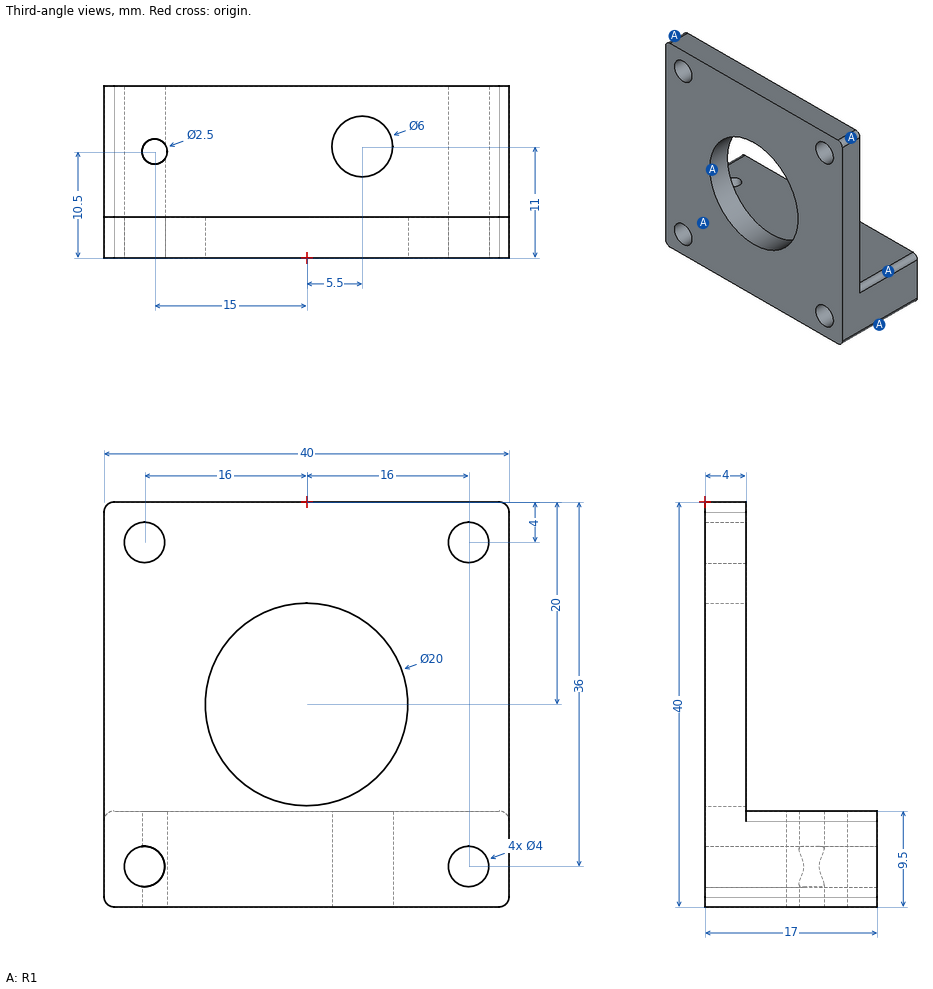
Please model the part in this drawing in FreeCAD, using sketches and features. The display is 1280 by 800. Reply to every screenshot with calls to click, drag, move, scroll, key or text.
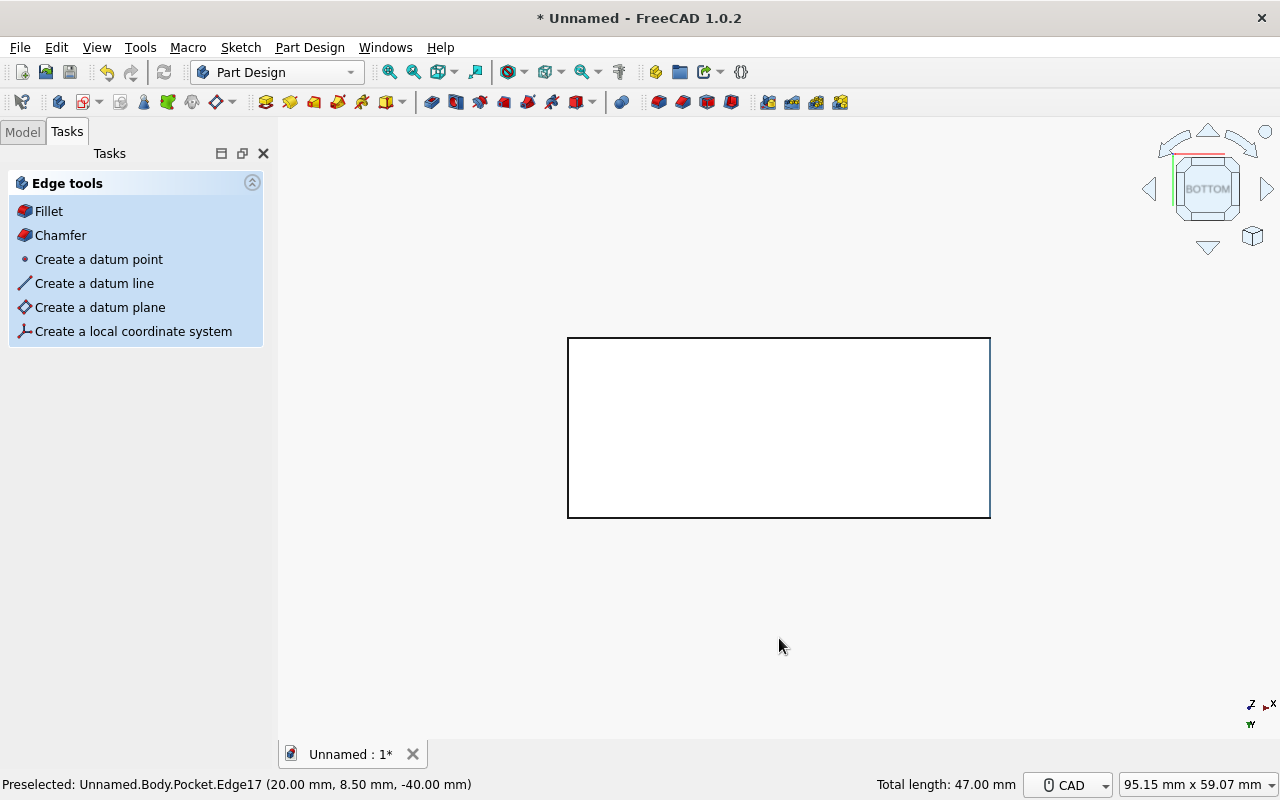
key(v)
key(f)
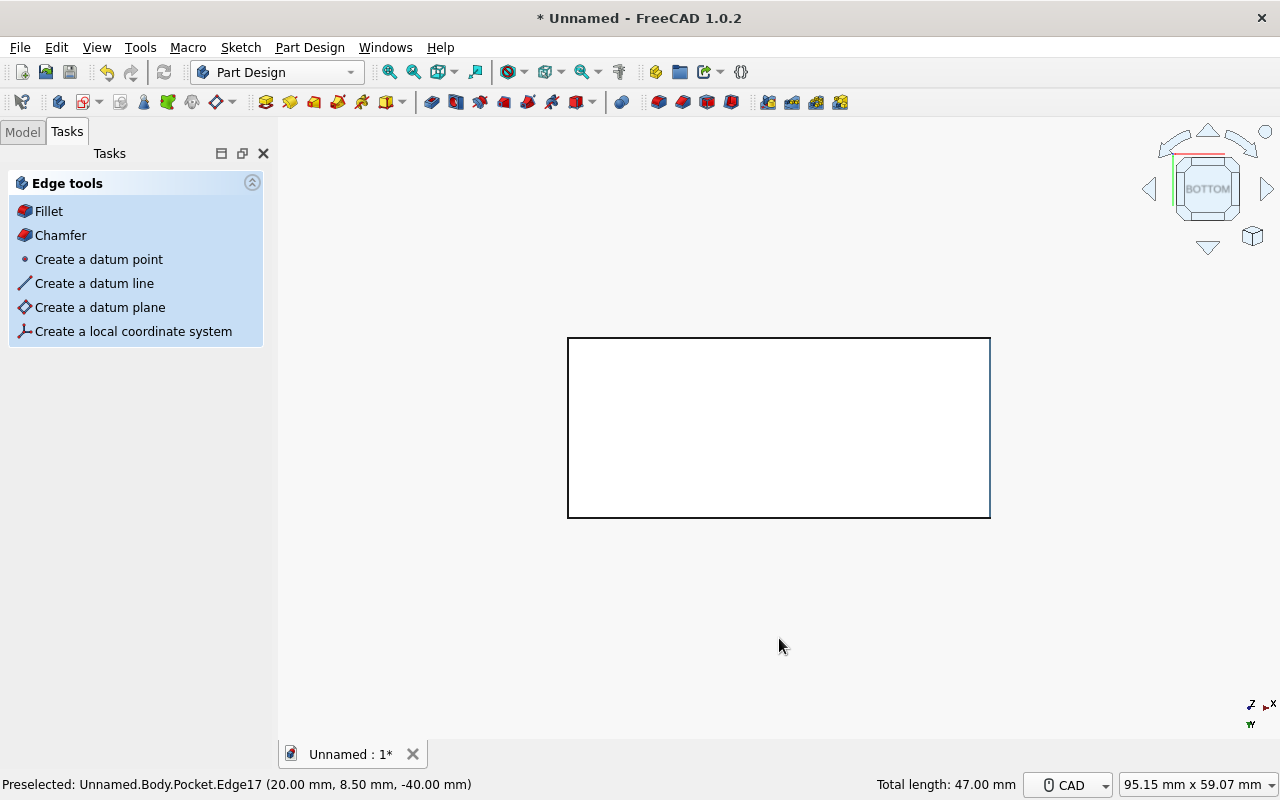
click(568, 427, ctrl)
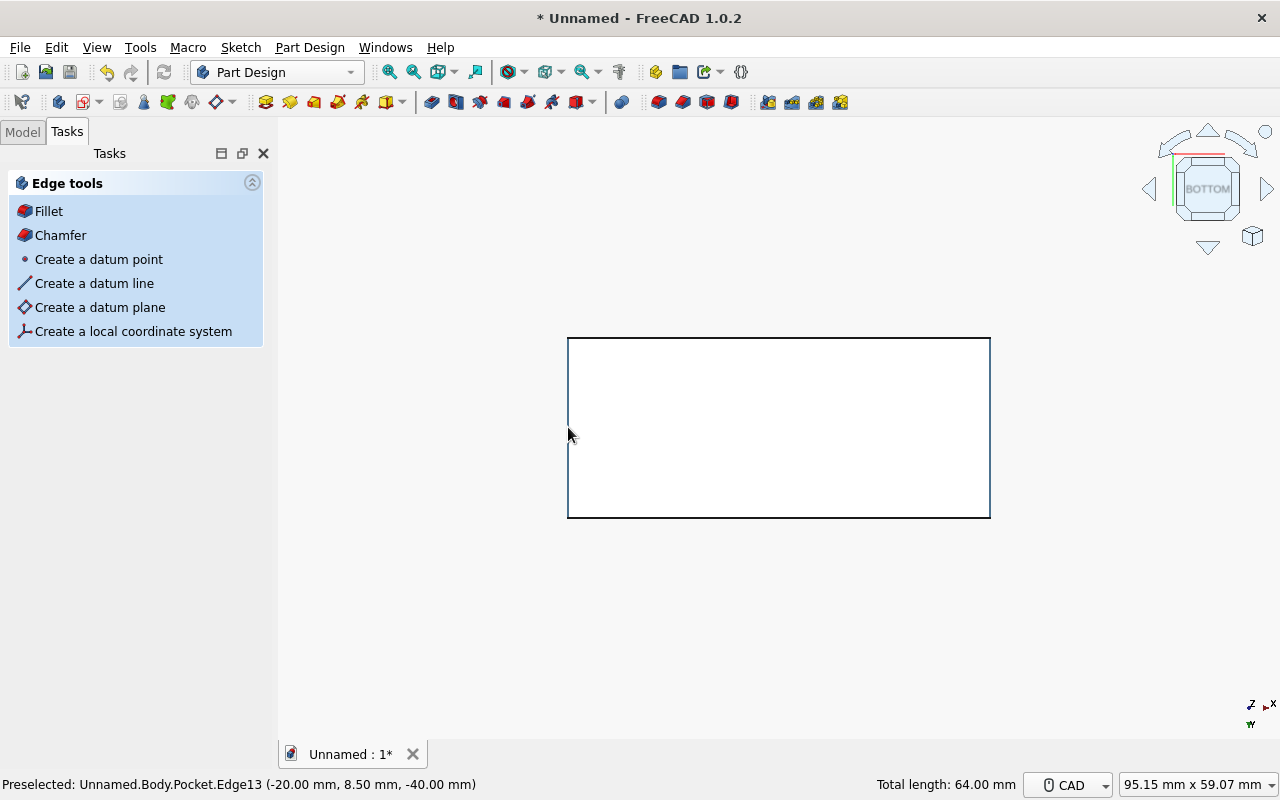
key(4)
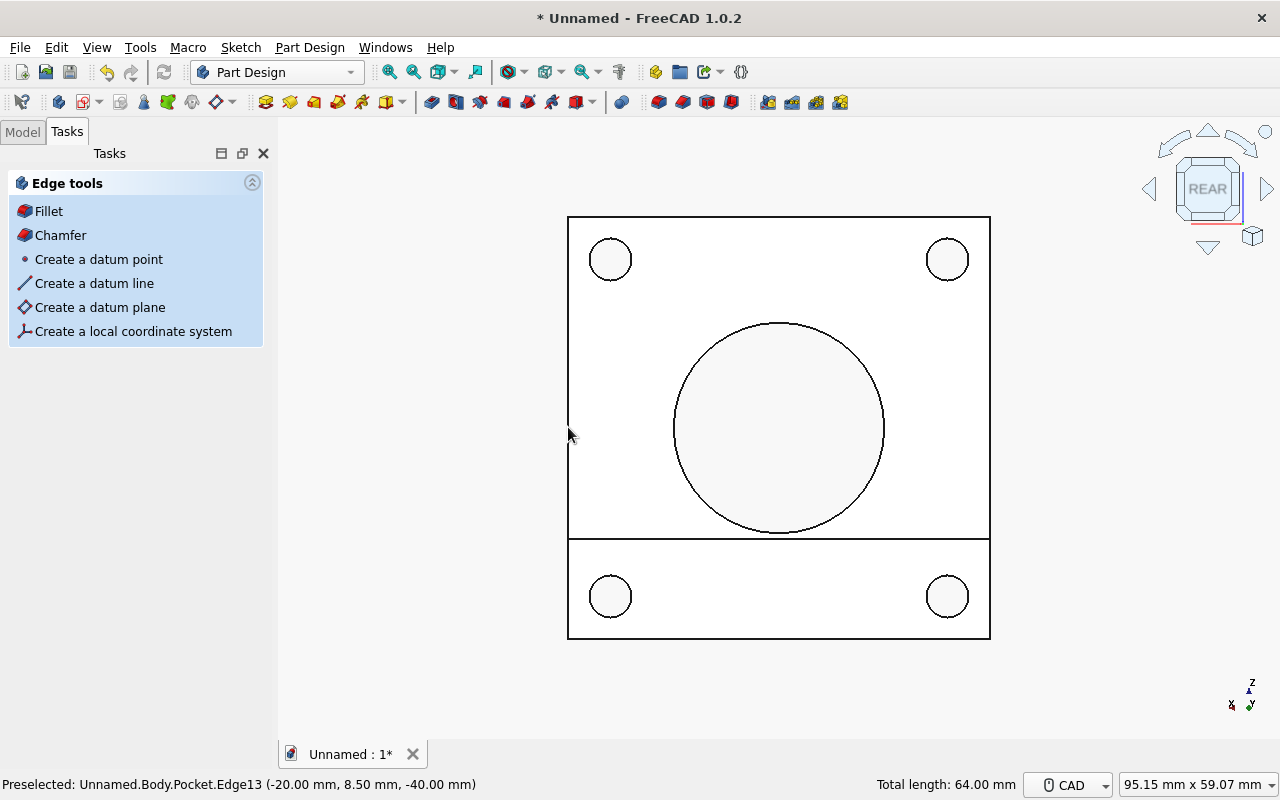
key(6)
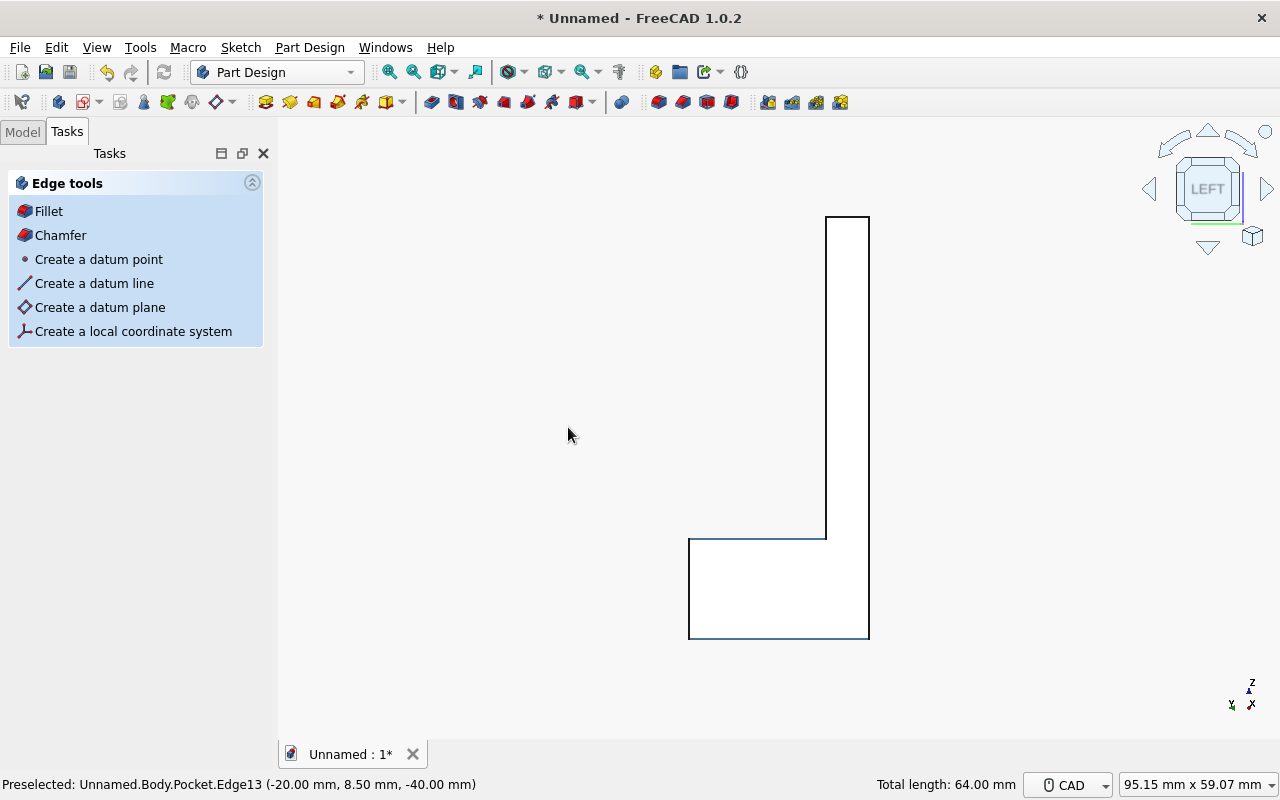
click(847, 216, ctrl)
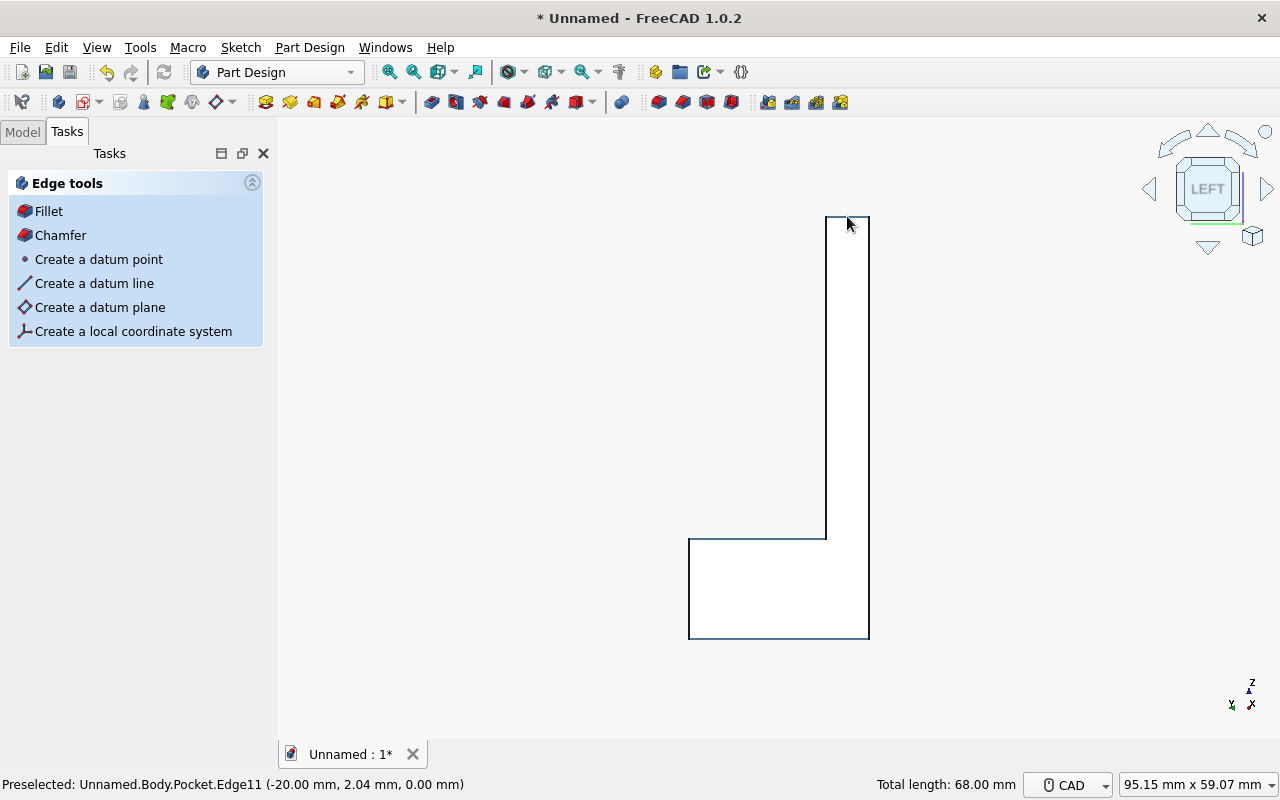
click(660, 102)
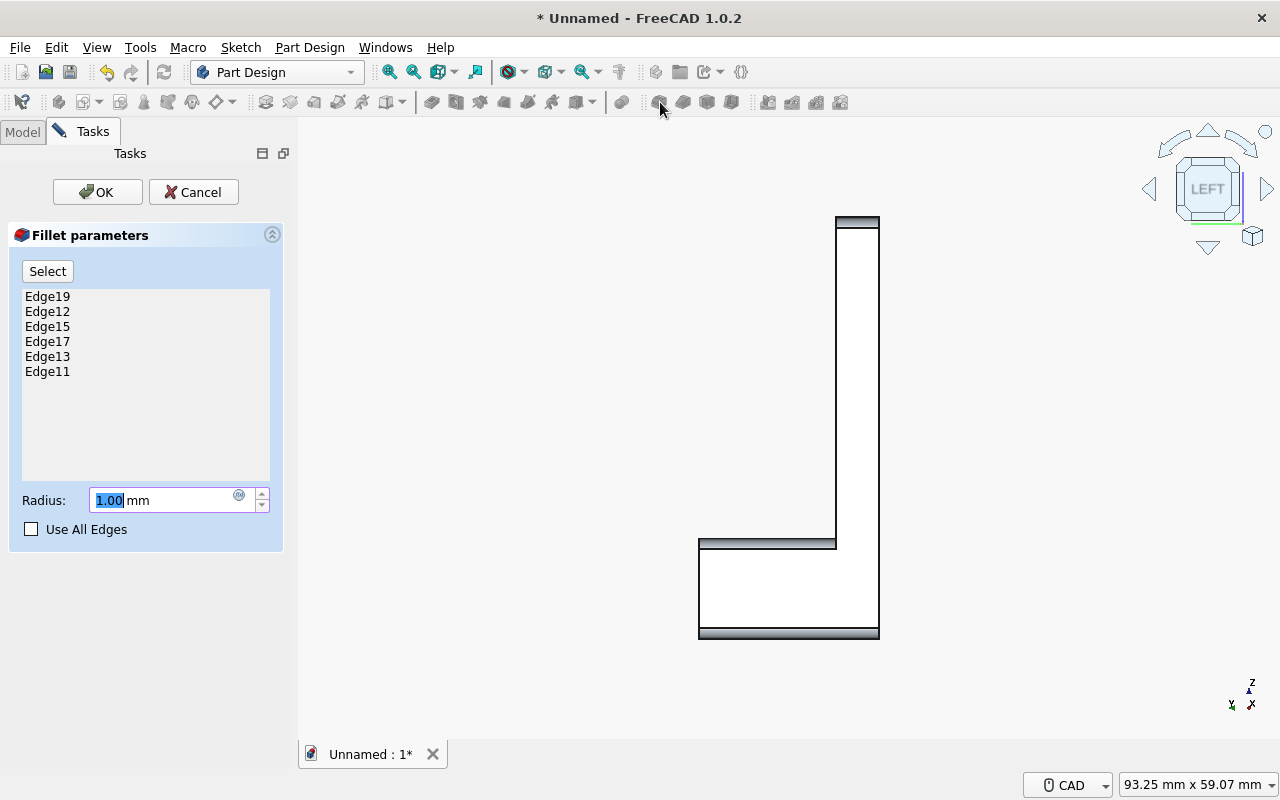
text(1)
key(Tab)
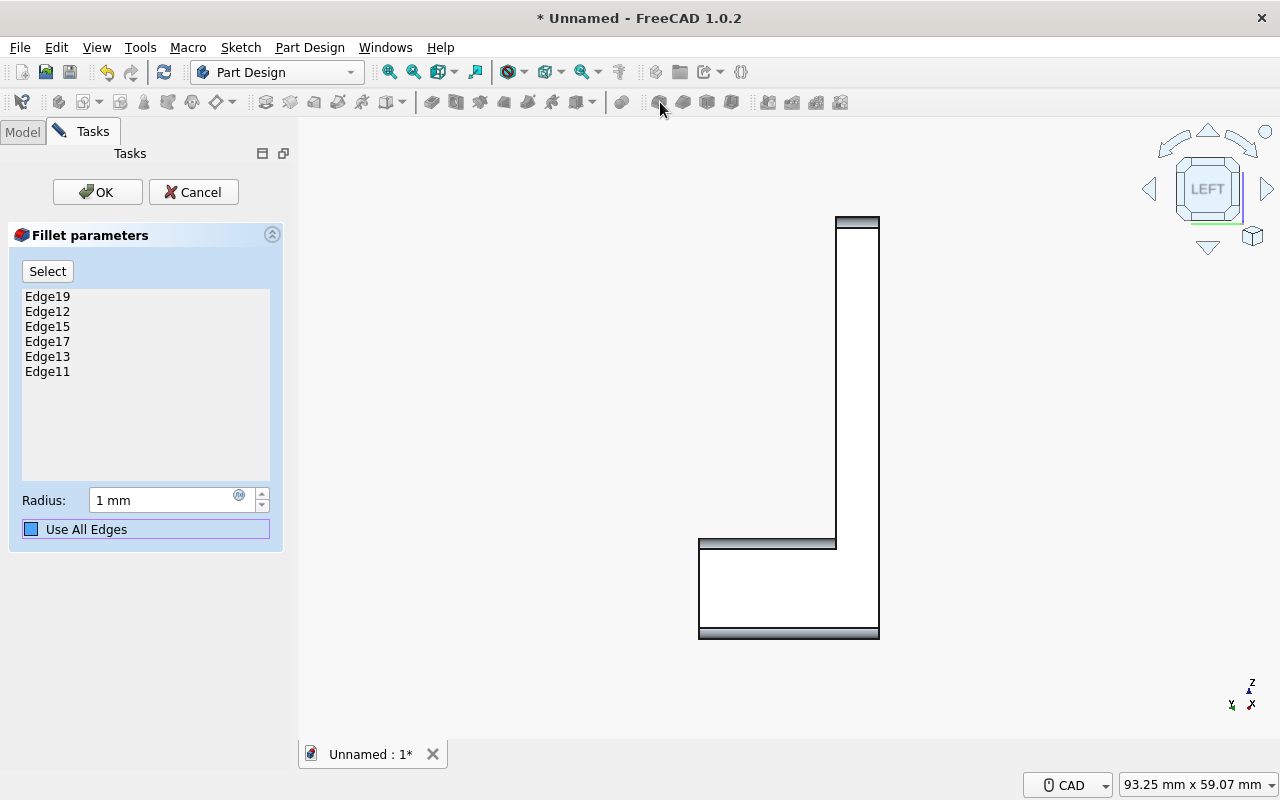
click(98, 192)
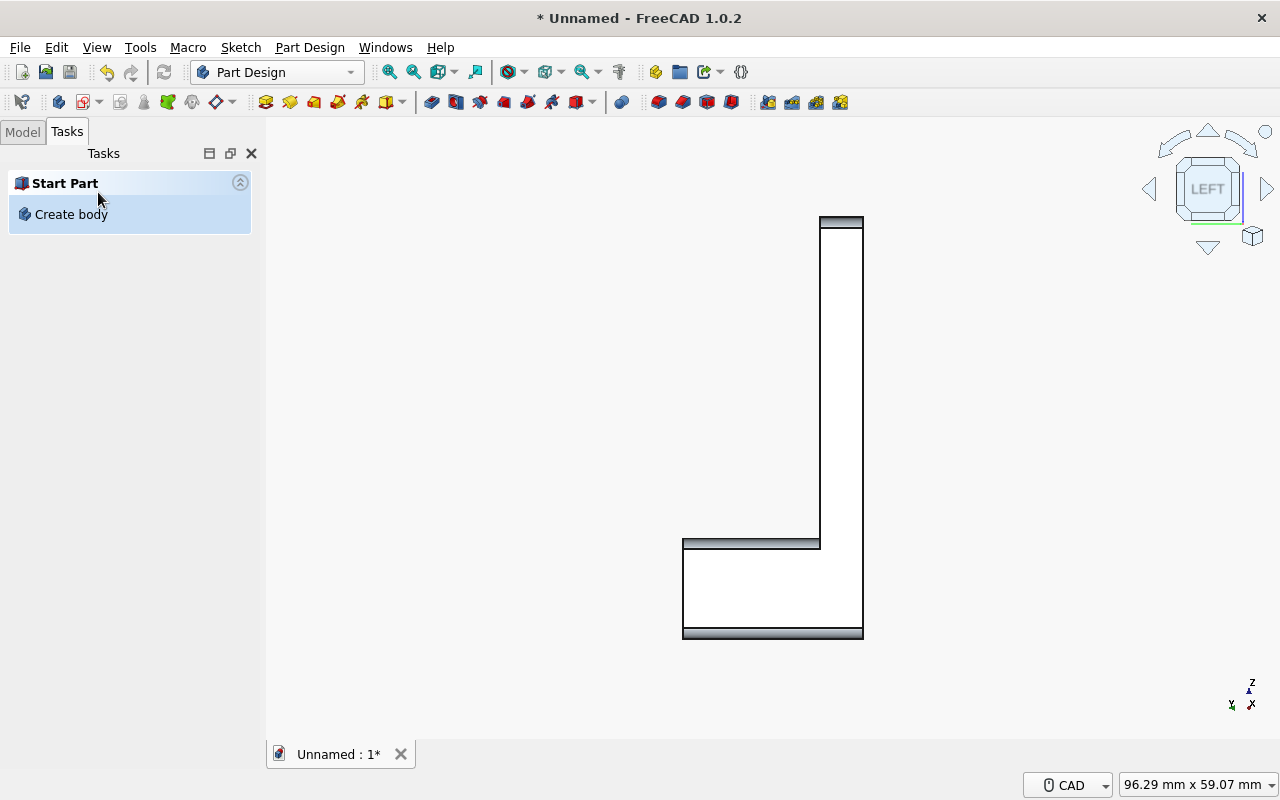
key(0)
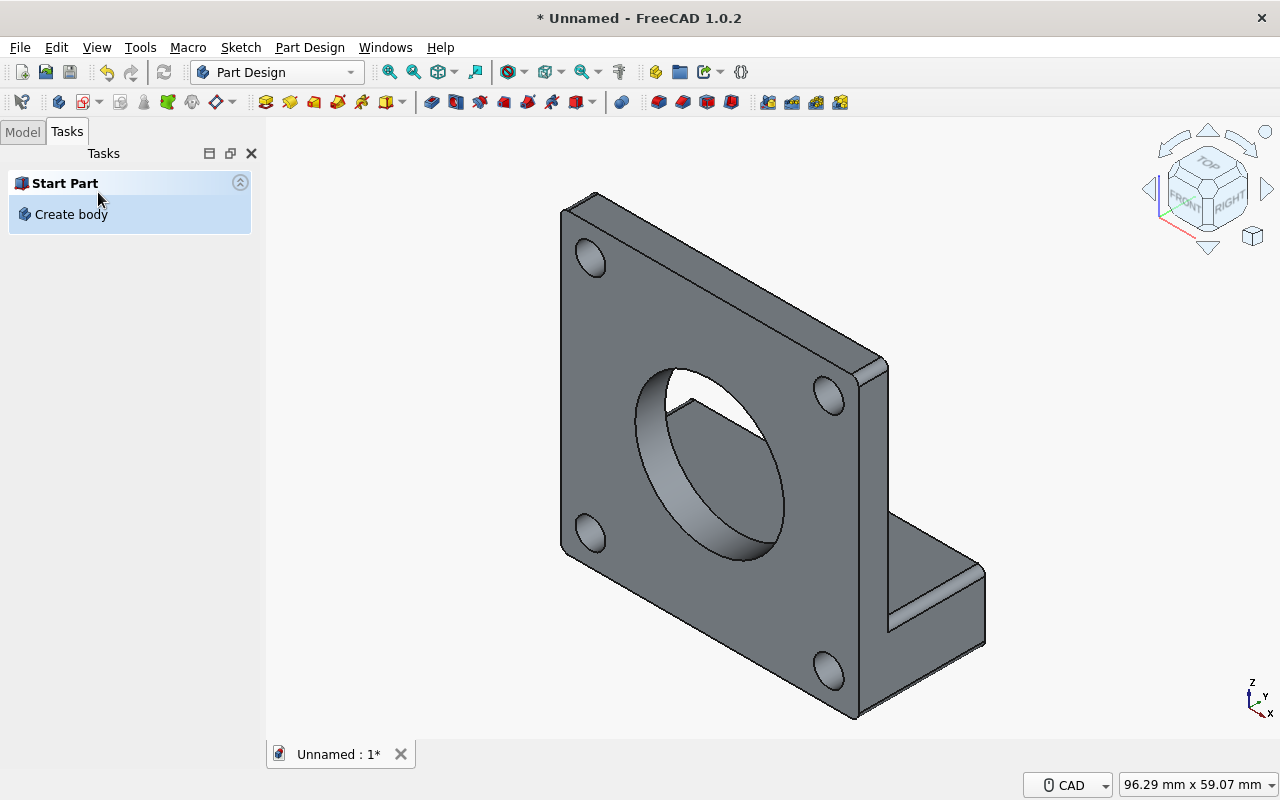
click(747, 485)